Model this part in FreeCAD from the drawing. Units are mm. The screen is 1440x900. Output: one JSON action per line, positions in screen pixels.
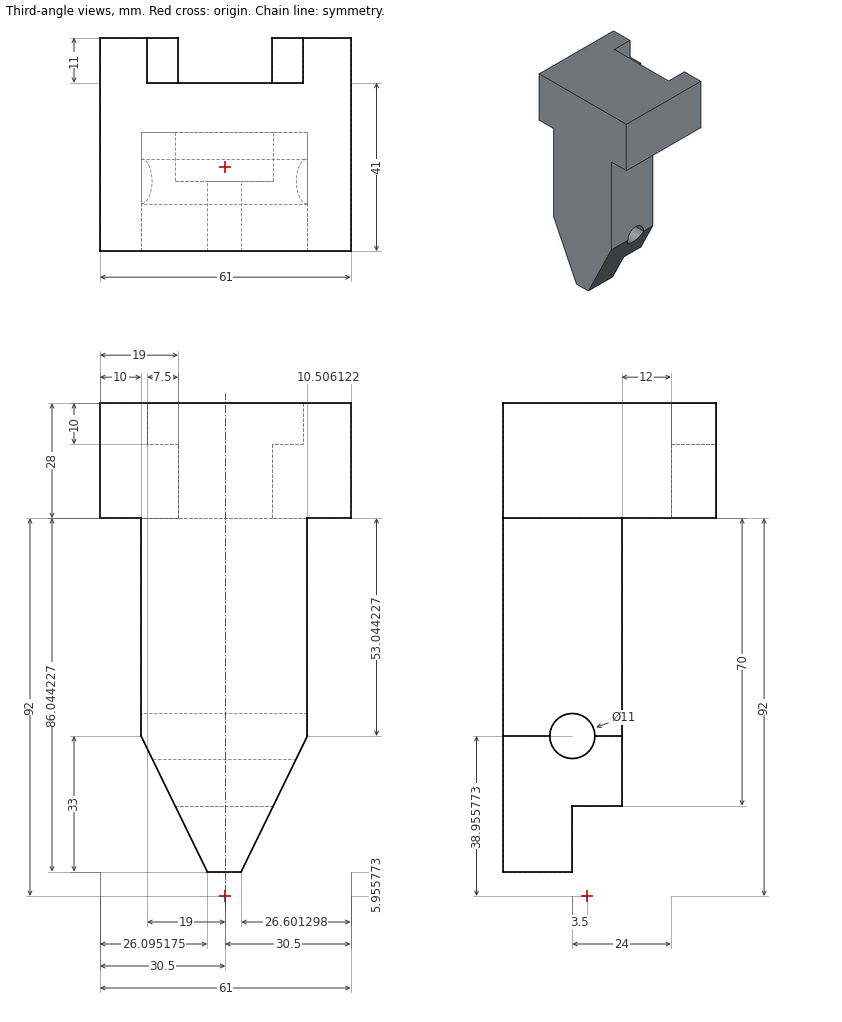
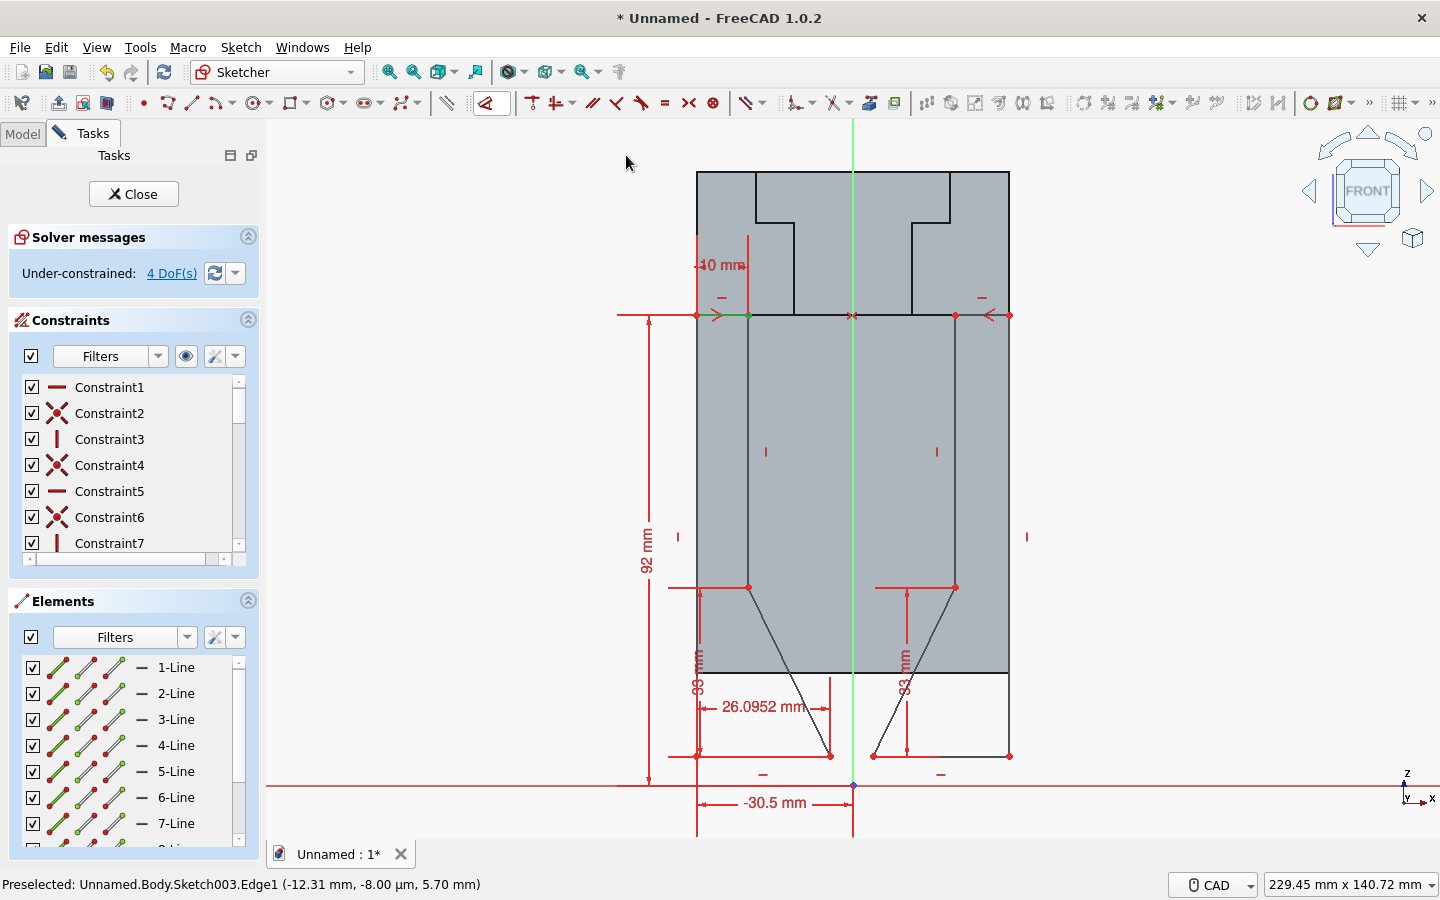
{"action": "left_click", "coordinate": [697, 624]}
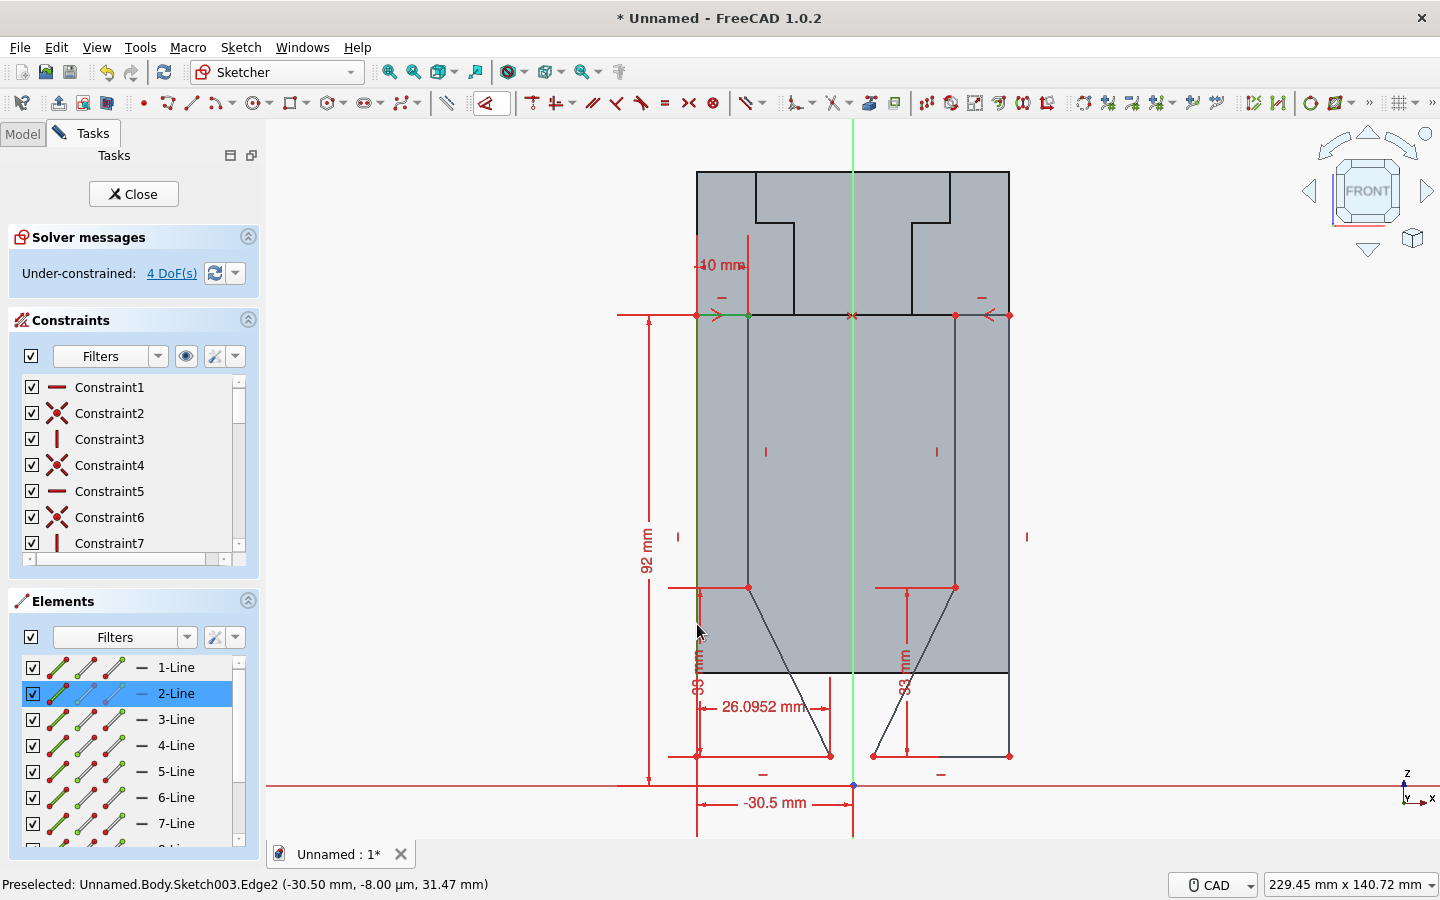
{"action": "left_click", "coordinate": [504, 104]}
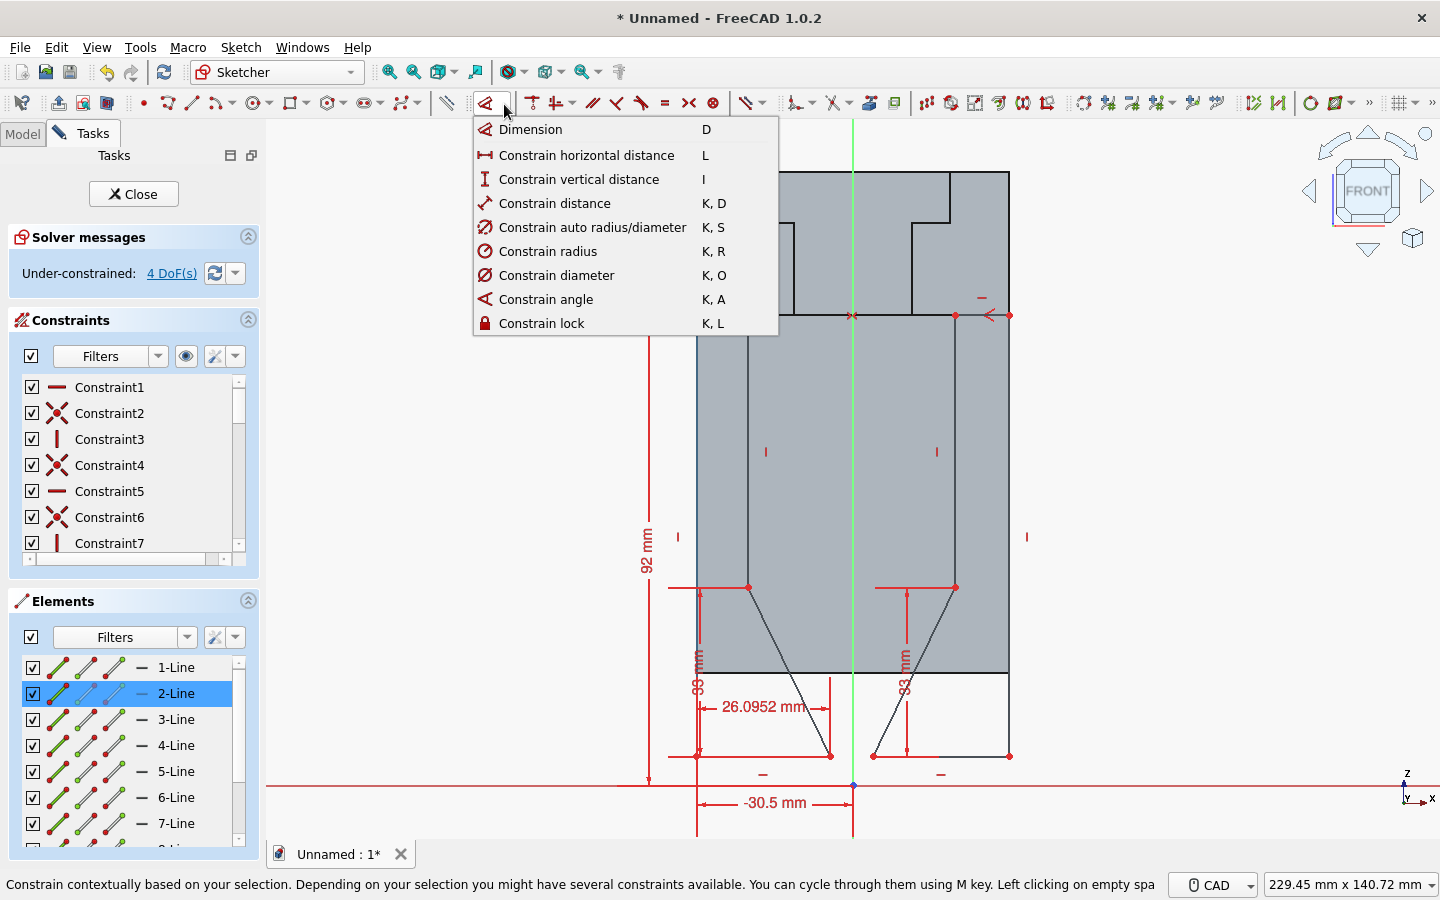
{"action": "left_click", "coordinate": [626, 179]}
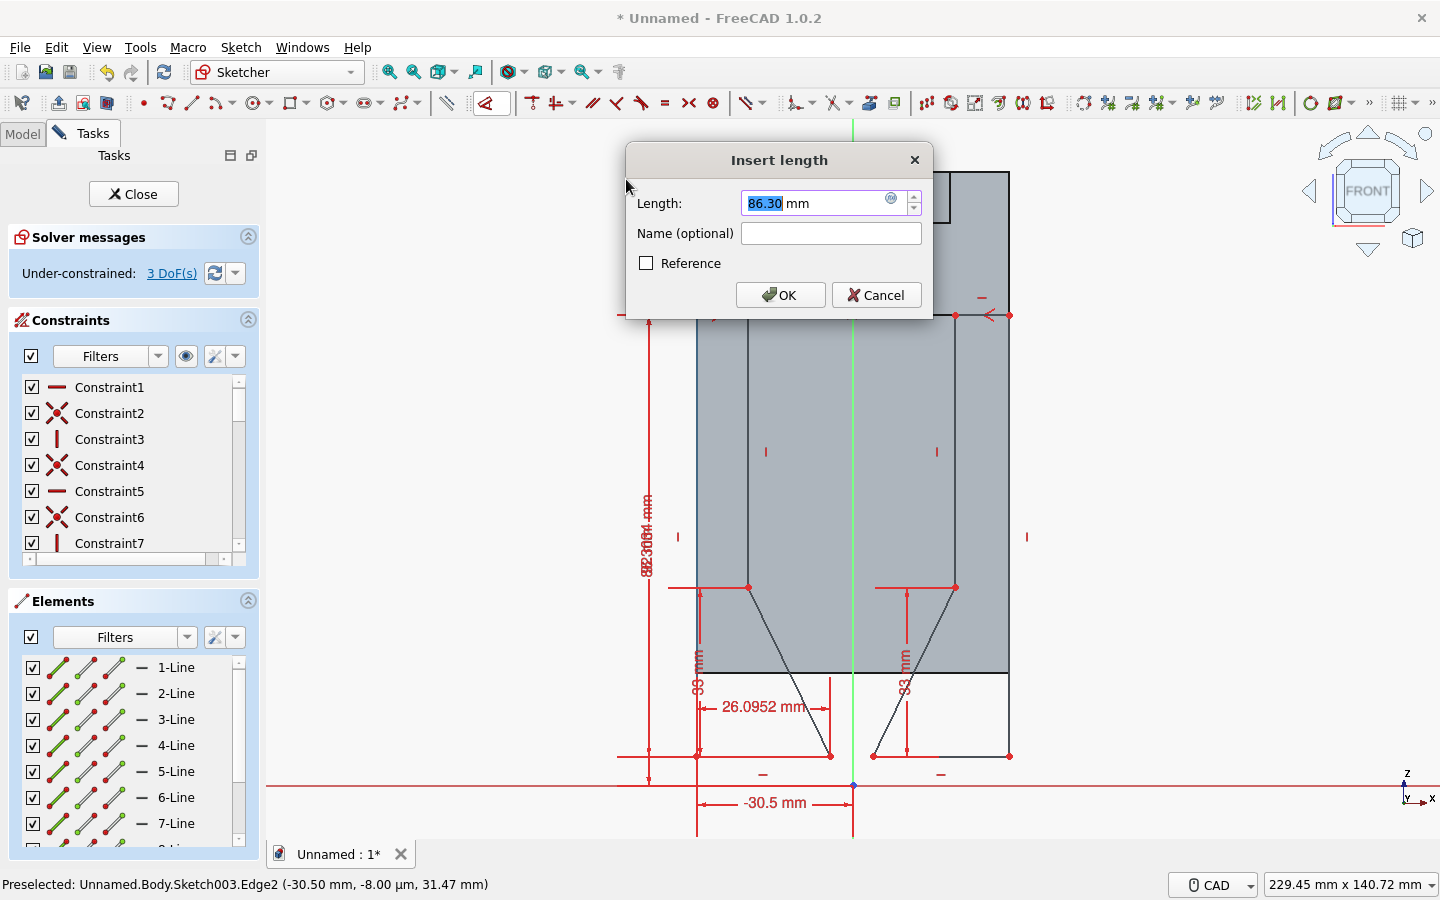
{"action": "type", "text": "86.044227"}
{"action": "key", "text": "Return"}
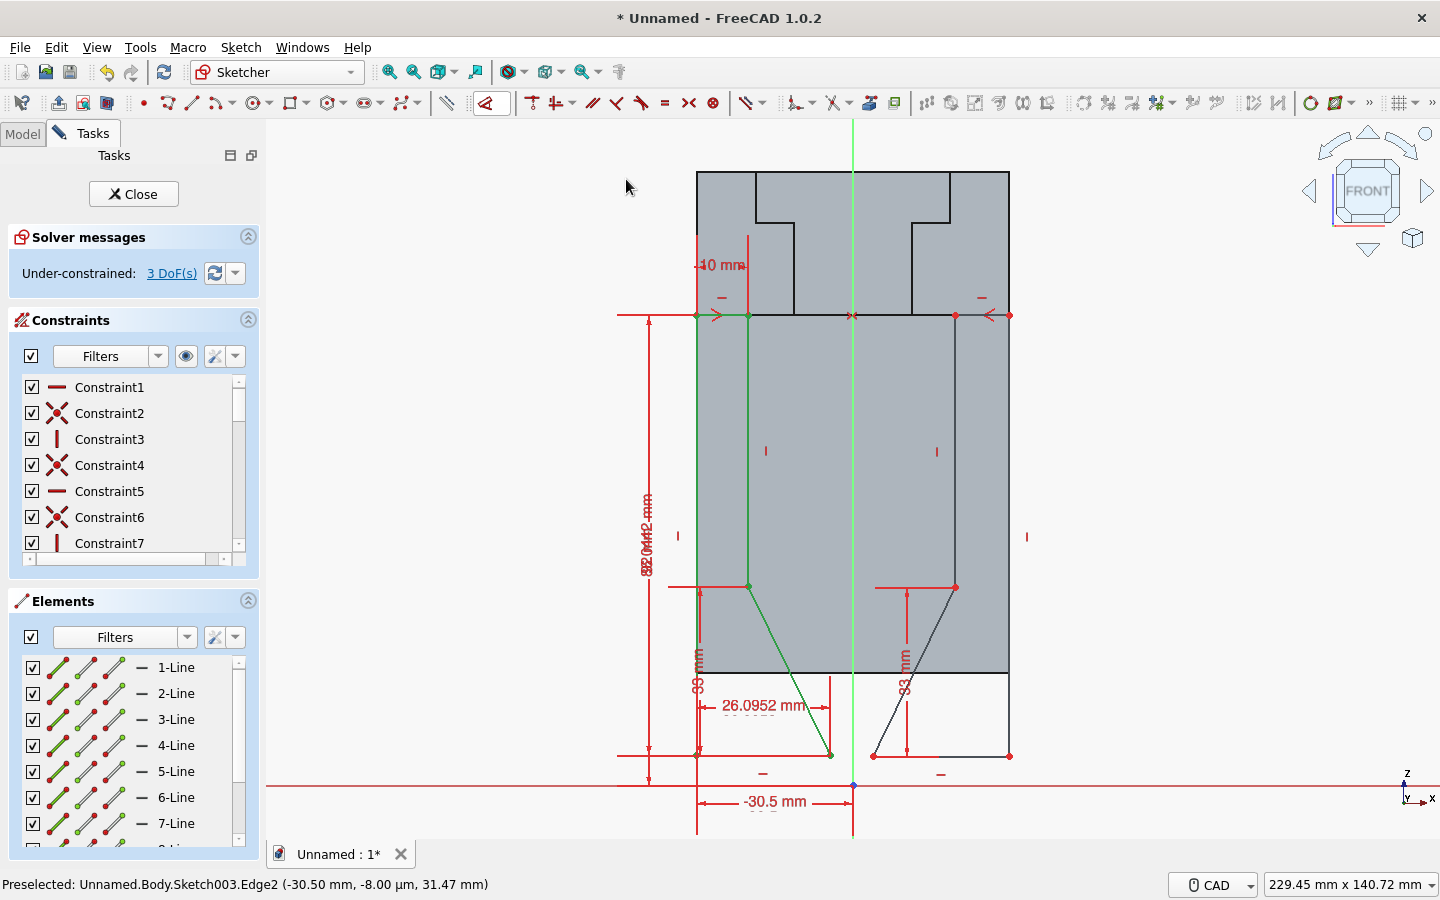
{"action": "left_click", "coordinate": [955, 506]}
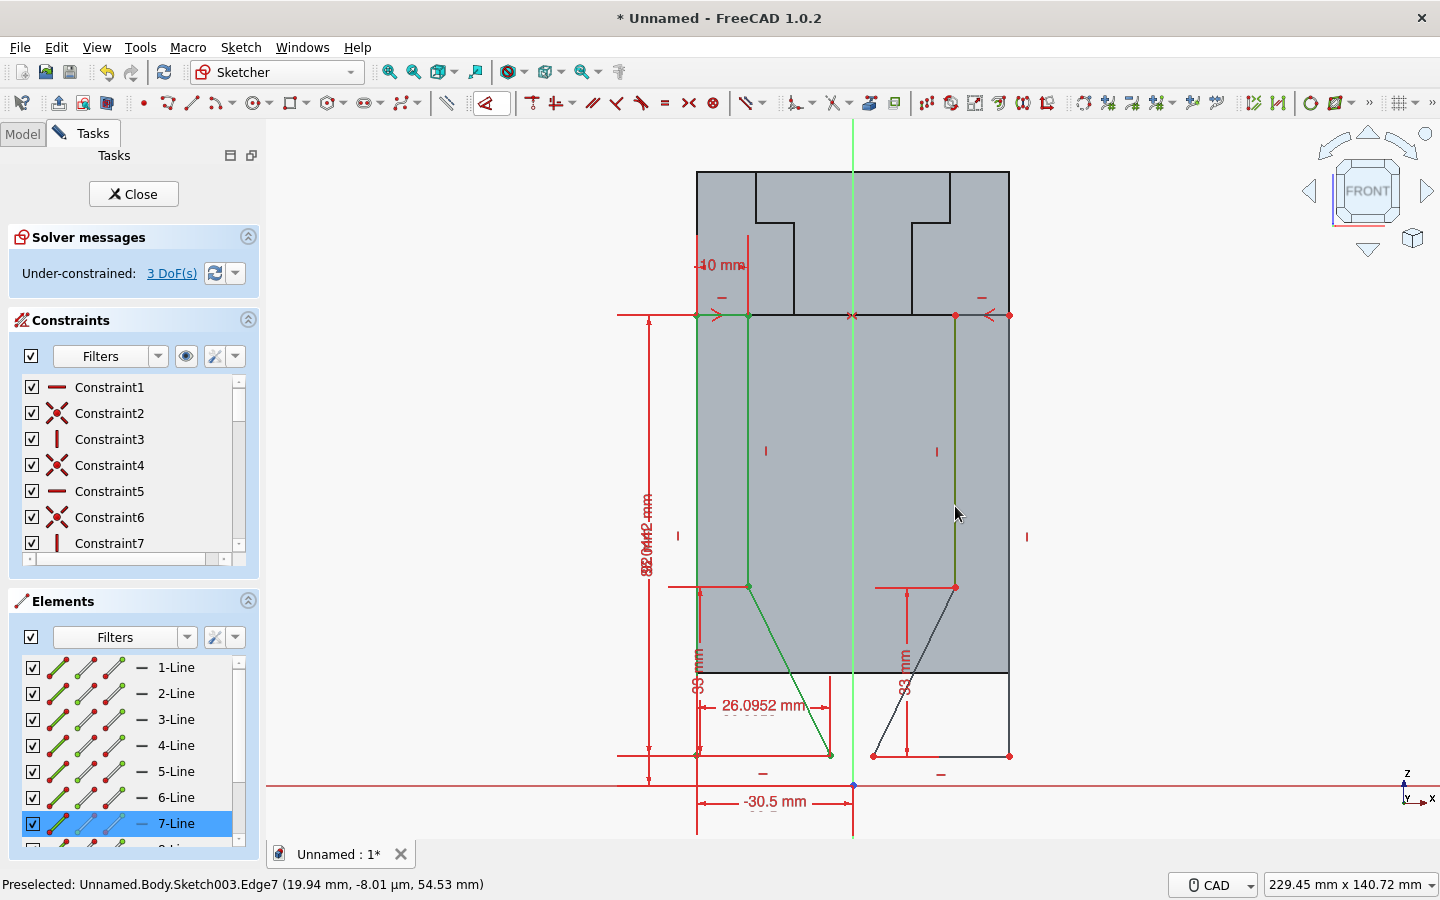
{"action": "key", "text": "i"}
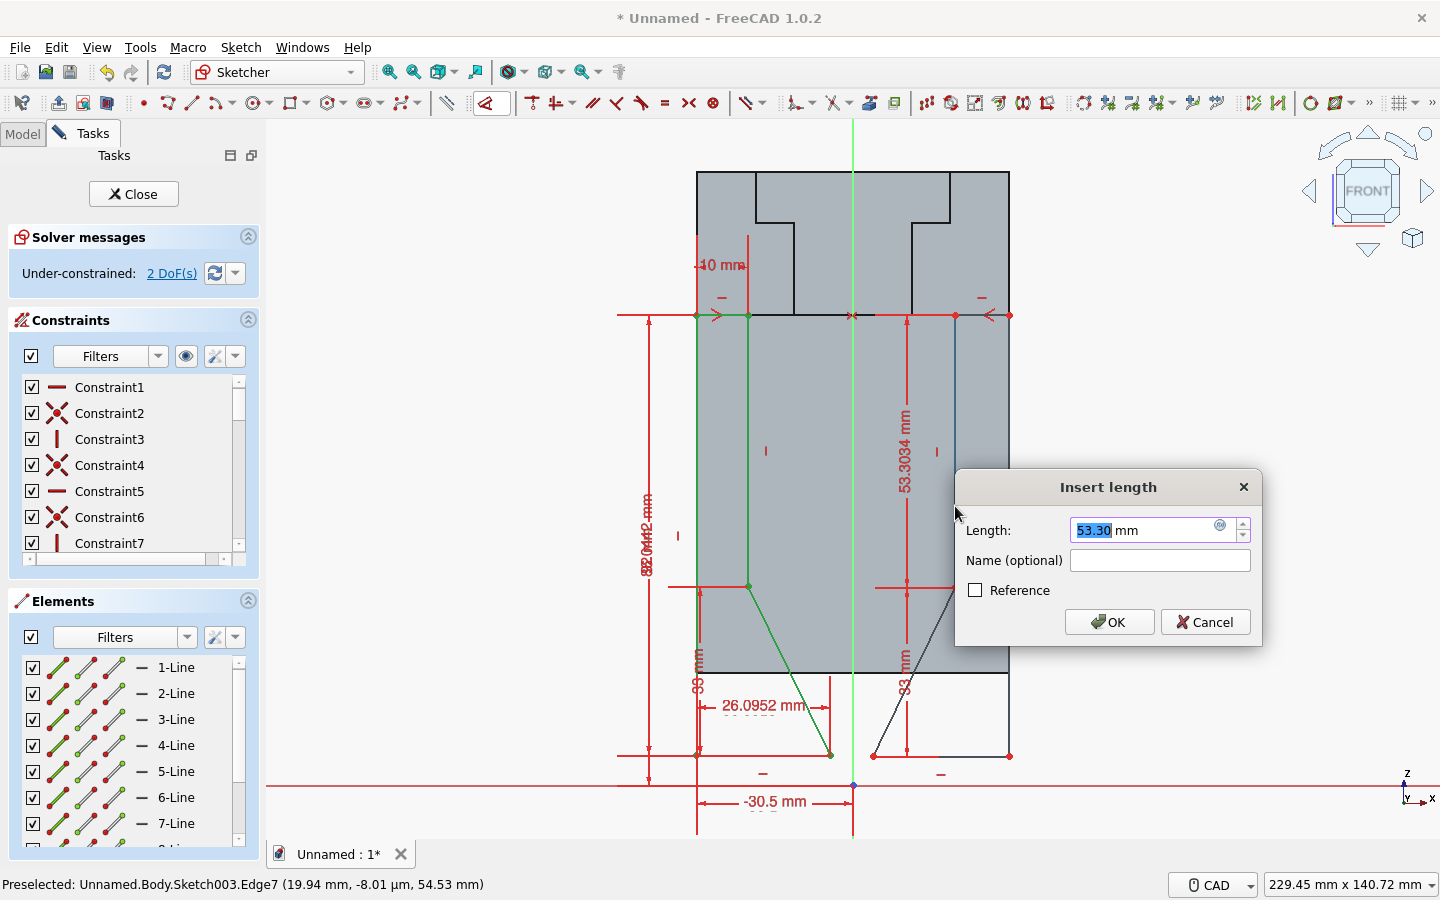
{"action": "type", "text": "53.044227"}
{"action": "key", "text": "Return"}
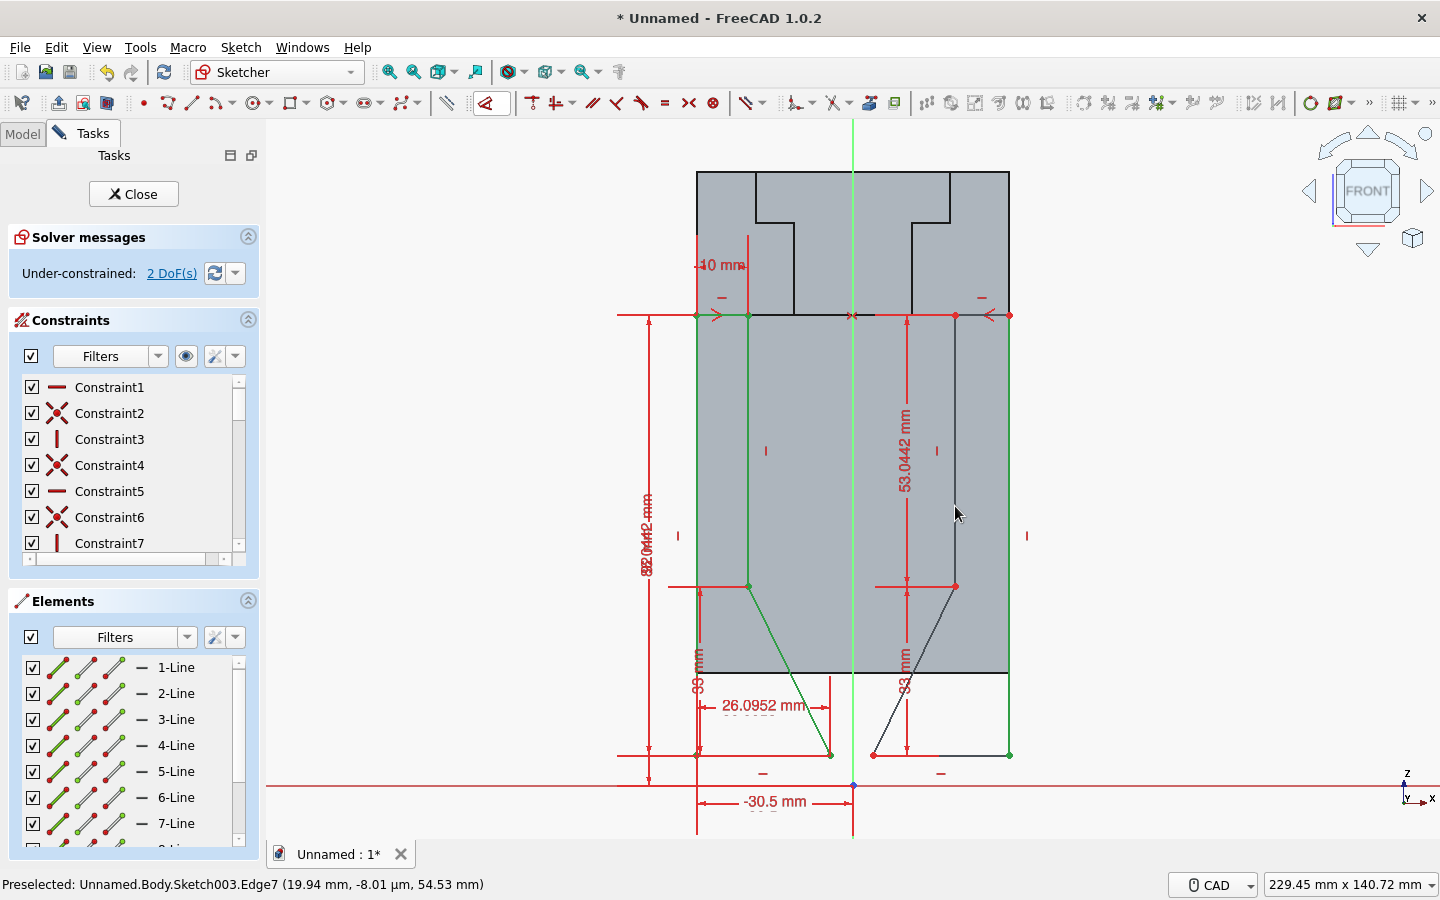
{"action": "left_click", "coordinate": [971, 315]}